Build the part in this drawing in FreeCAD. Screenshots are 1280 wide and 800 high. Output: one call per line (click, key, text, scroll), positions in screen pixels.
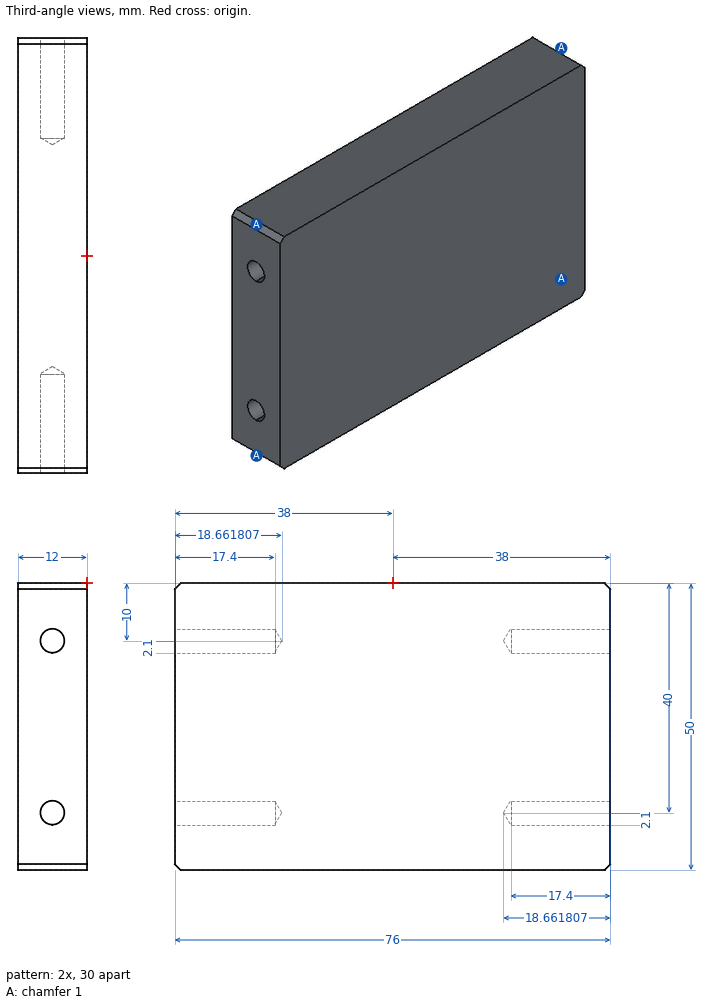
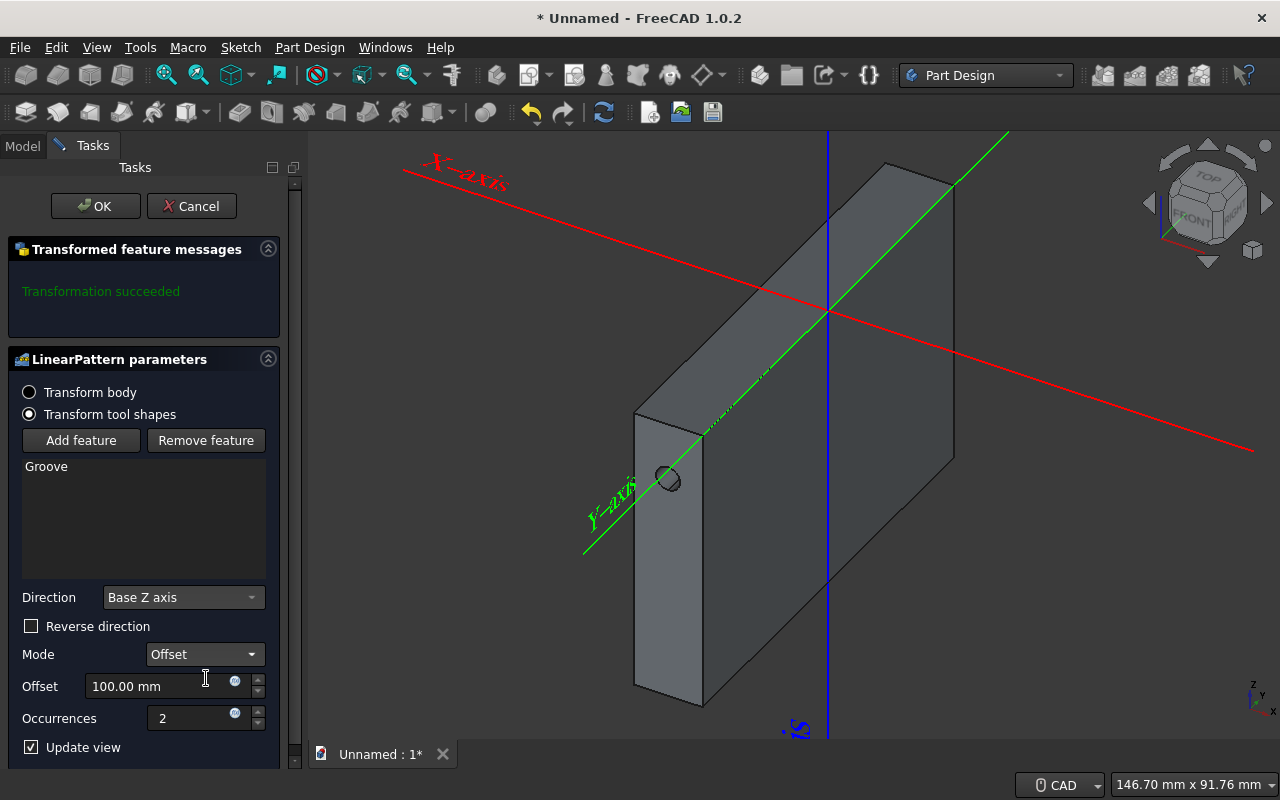
triple_click(168, 686)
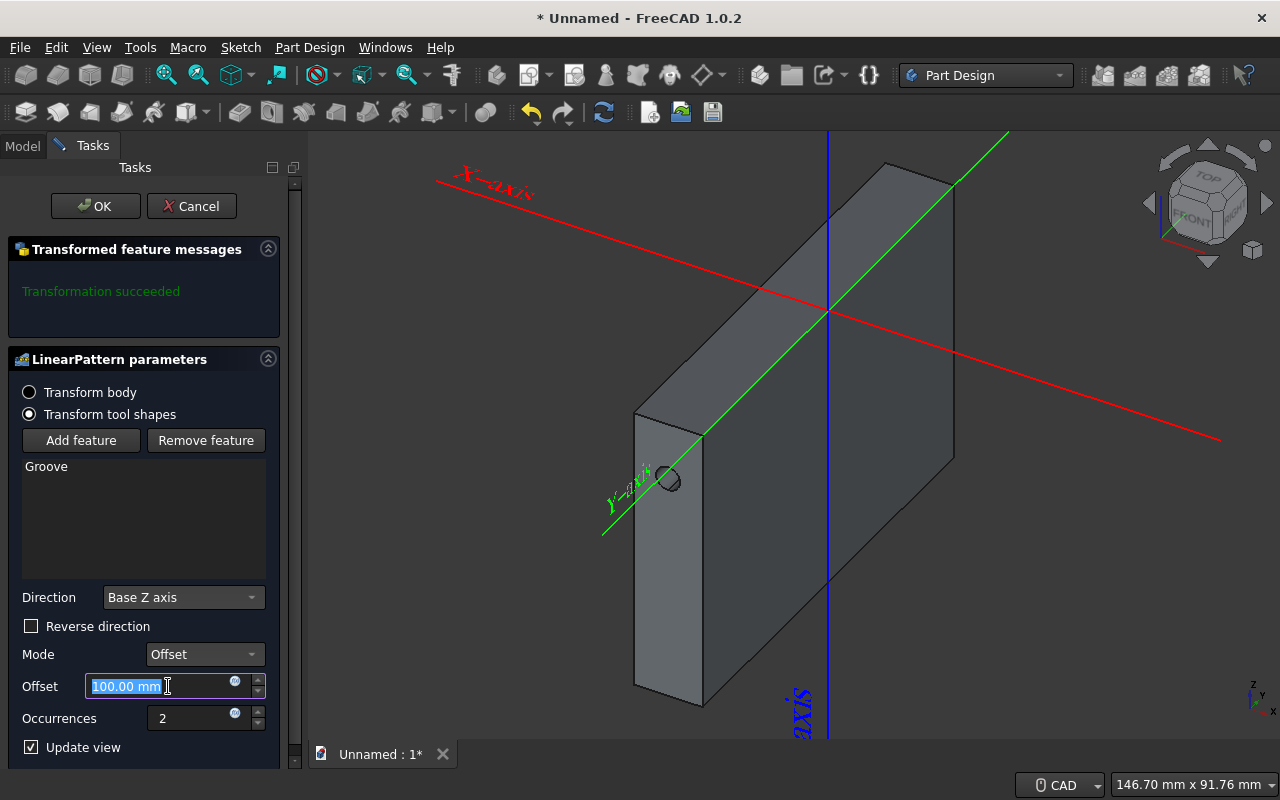
text(30)
key(Tab)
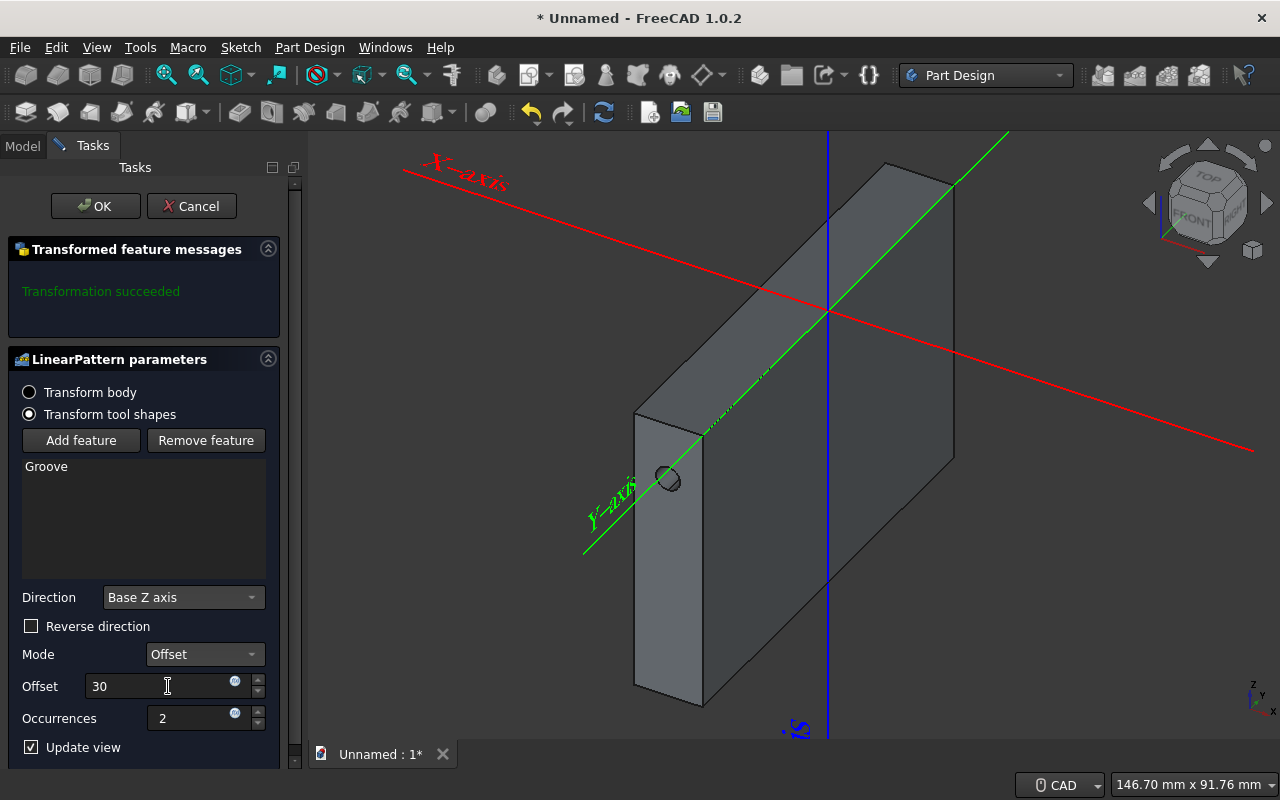
triple_click(198, 718)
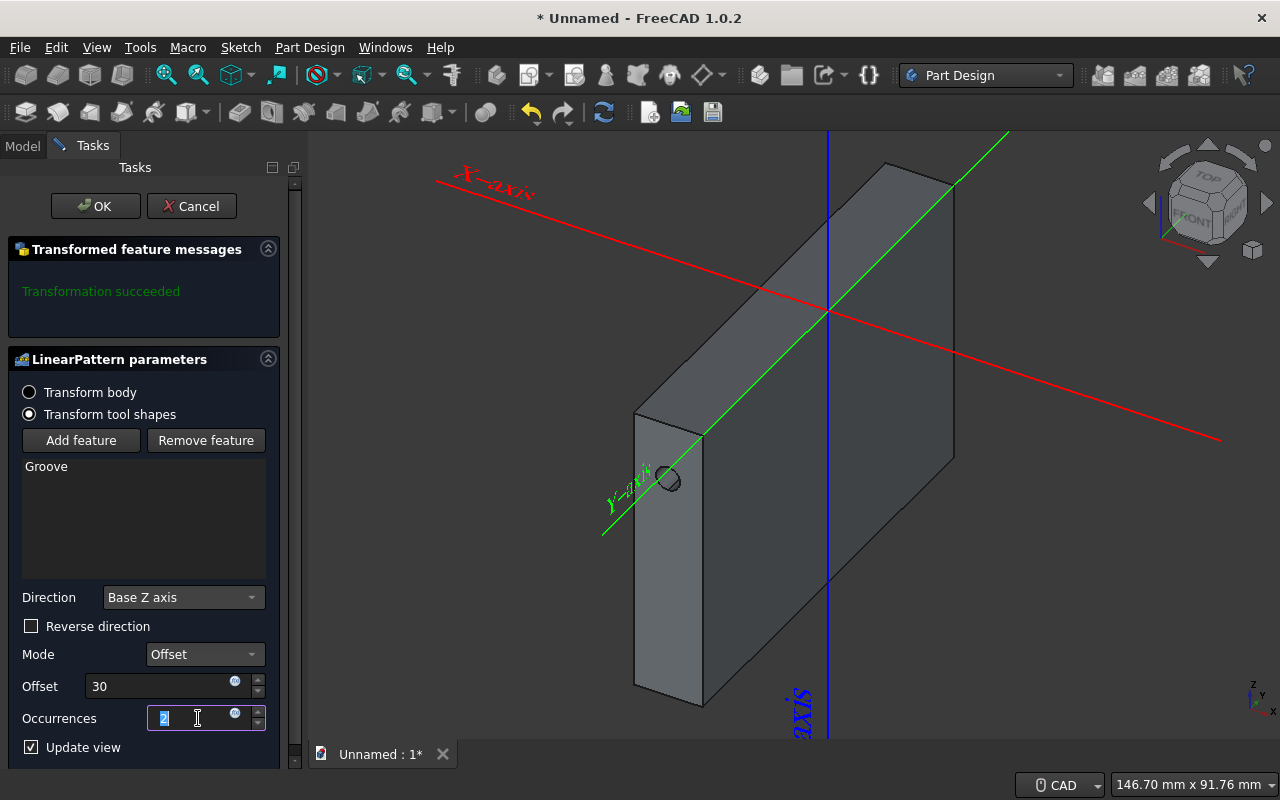
text(2)
key(Tab)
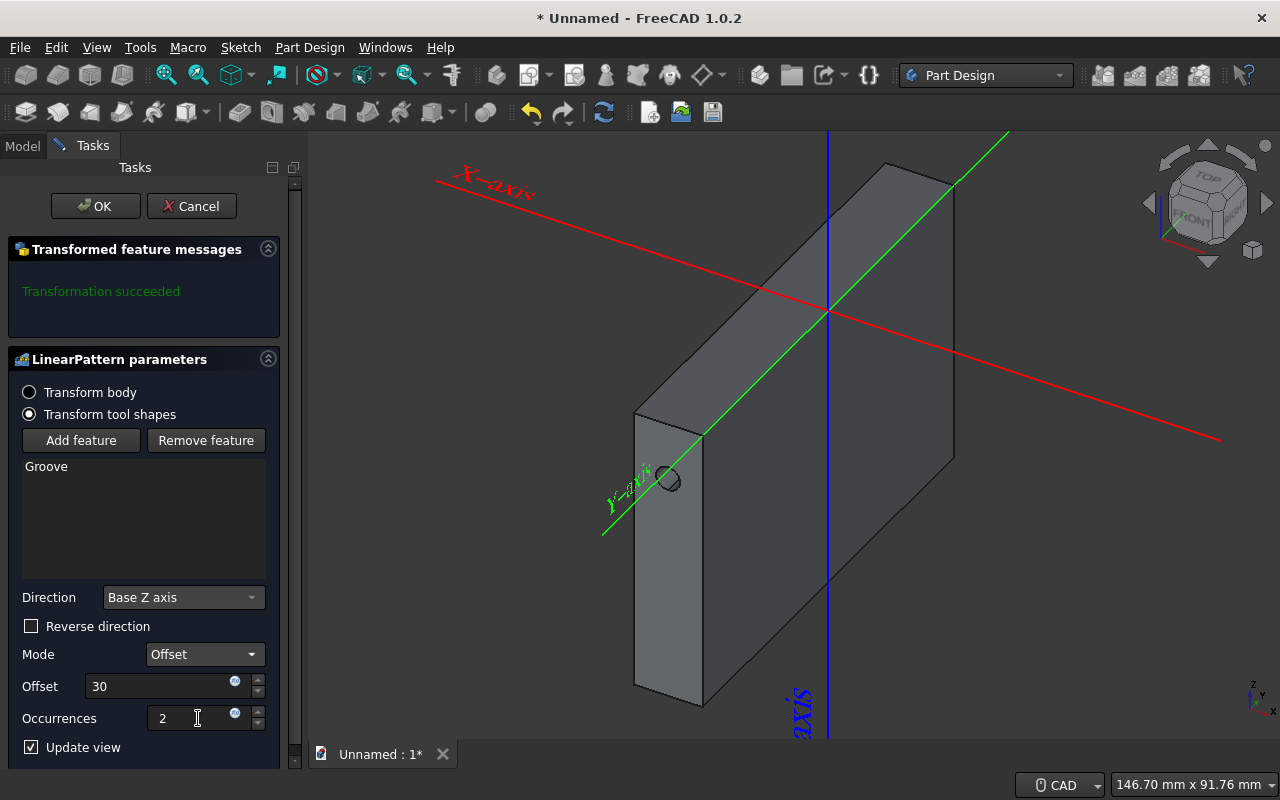
click(30, 626)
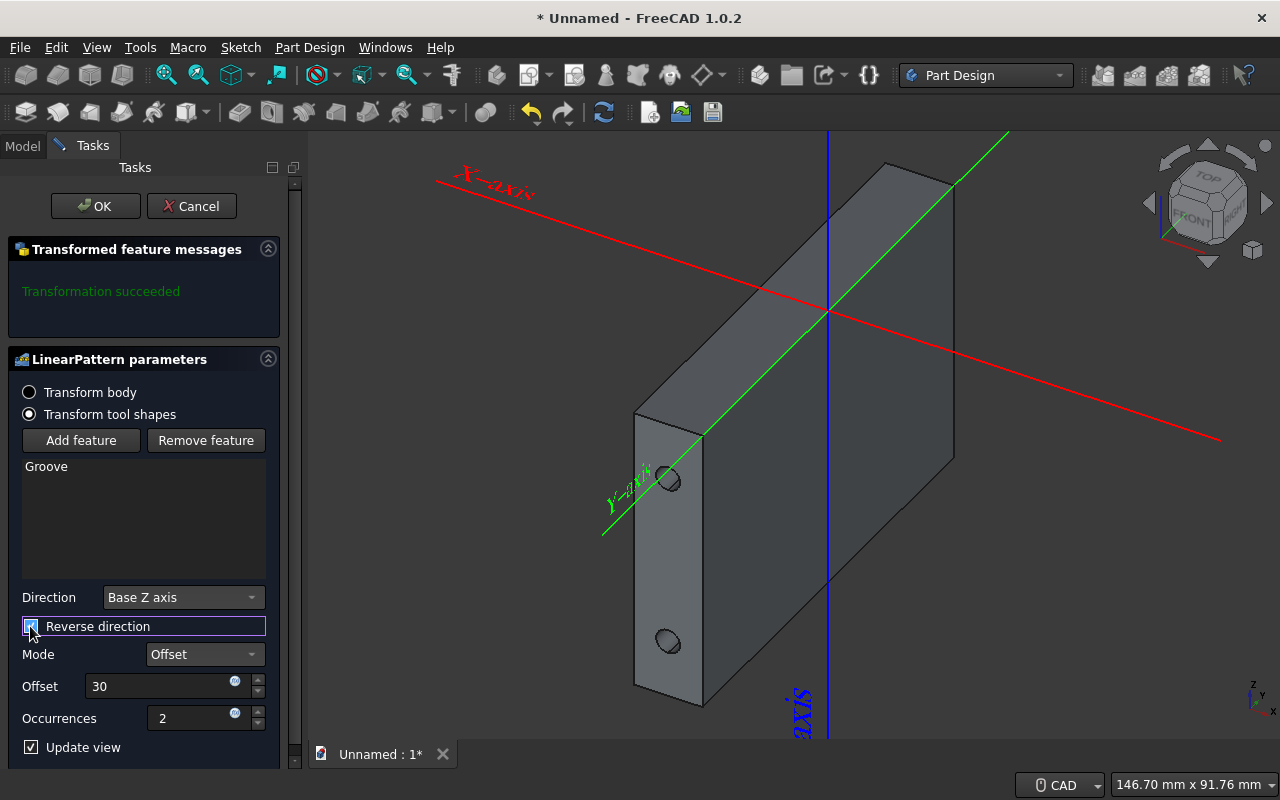
click(96, 206)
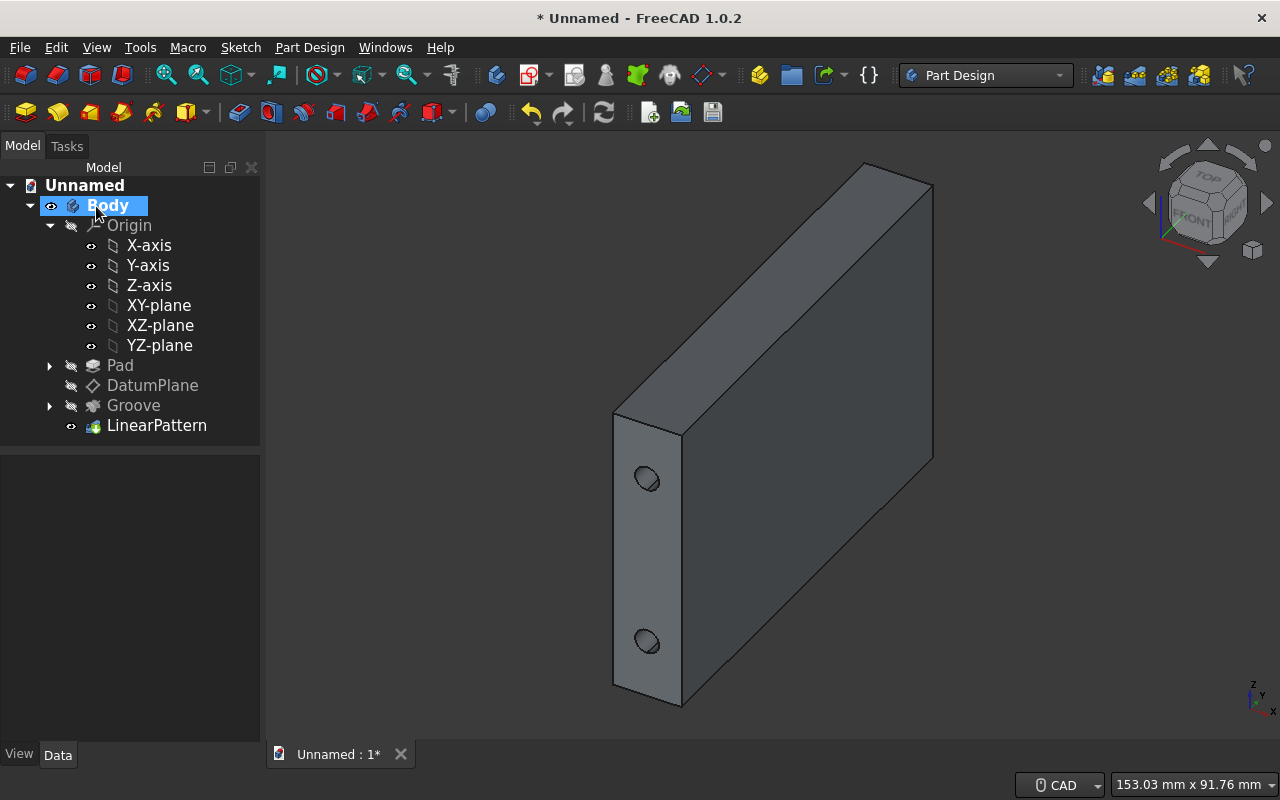
click(116, 406)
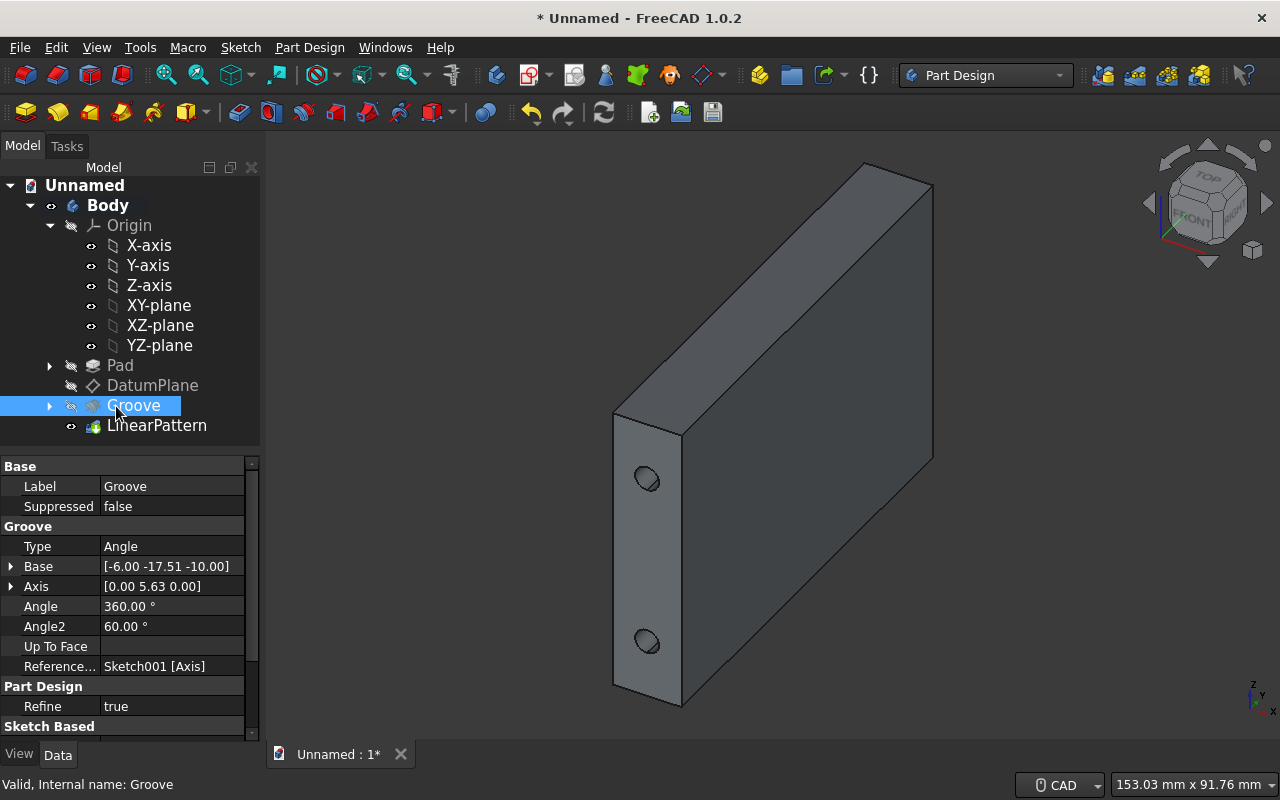
click(1104, 76)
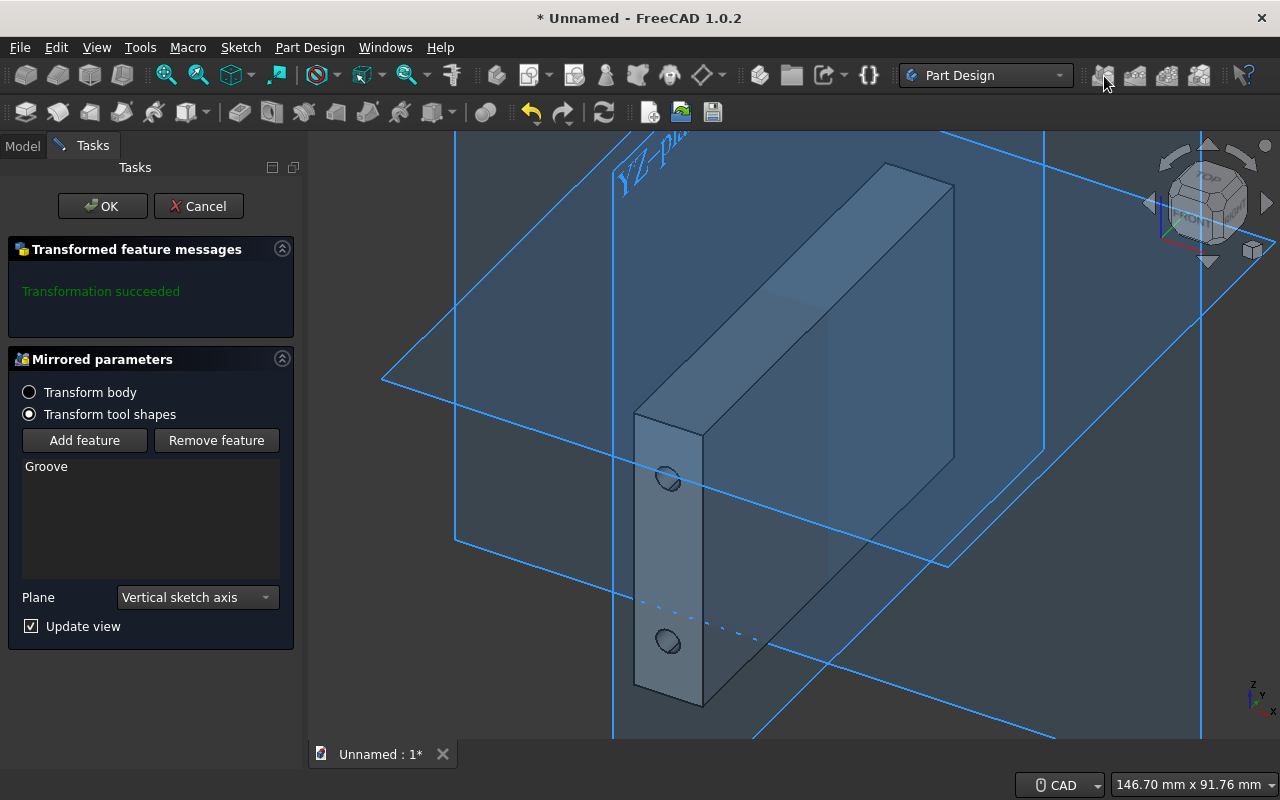
click(198, 598)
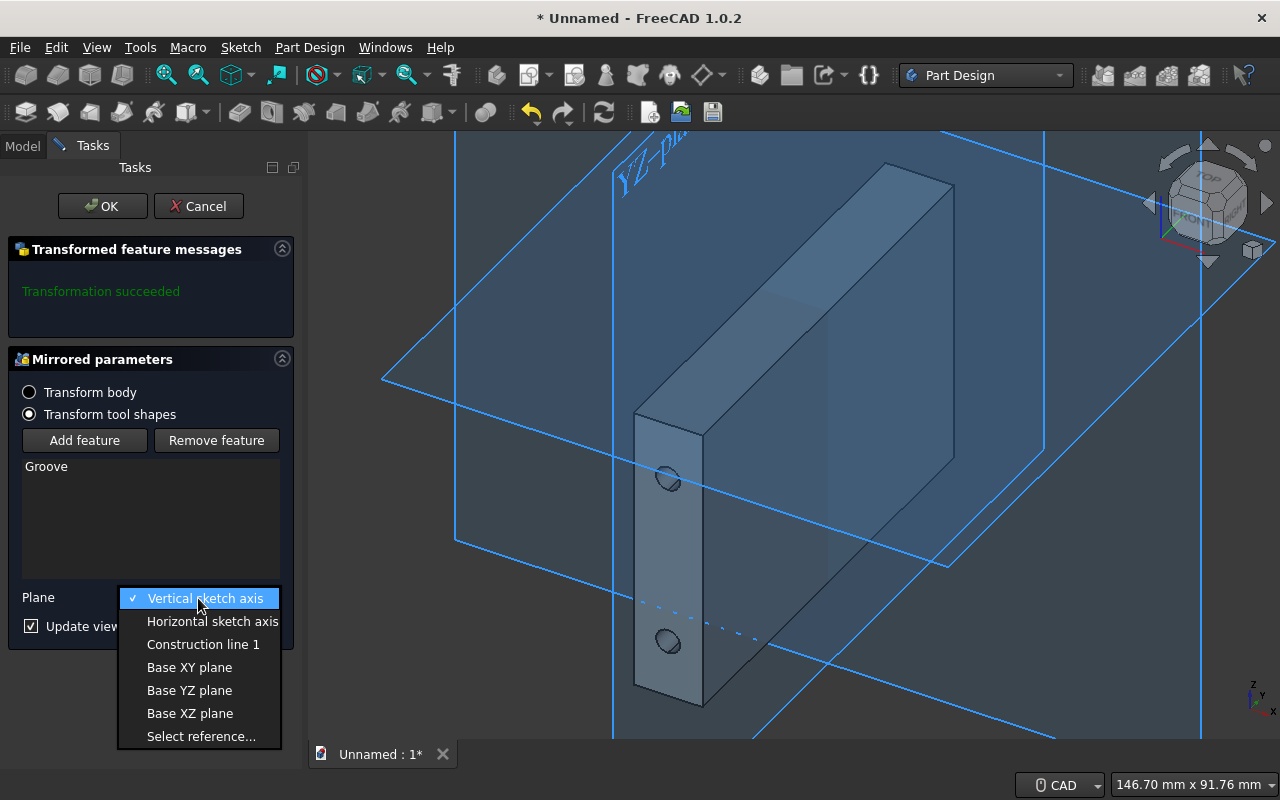
click(198, 714)